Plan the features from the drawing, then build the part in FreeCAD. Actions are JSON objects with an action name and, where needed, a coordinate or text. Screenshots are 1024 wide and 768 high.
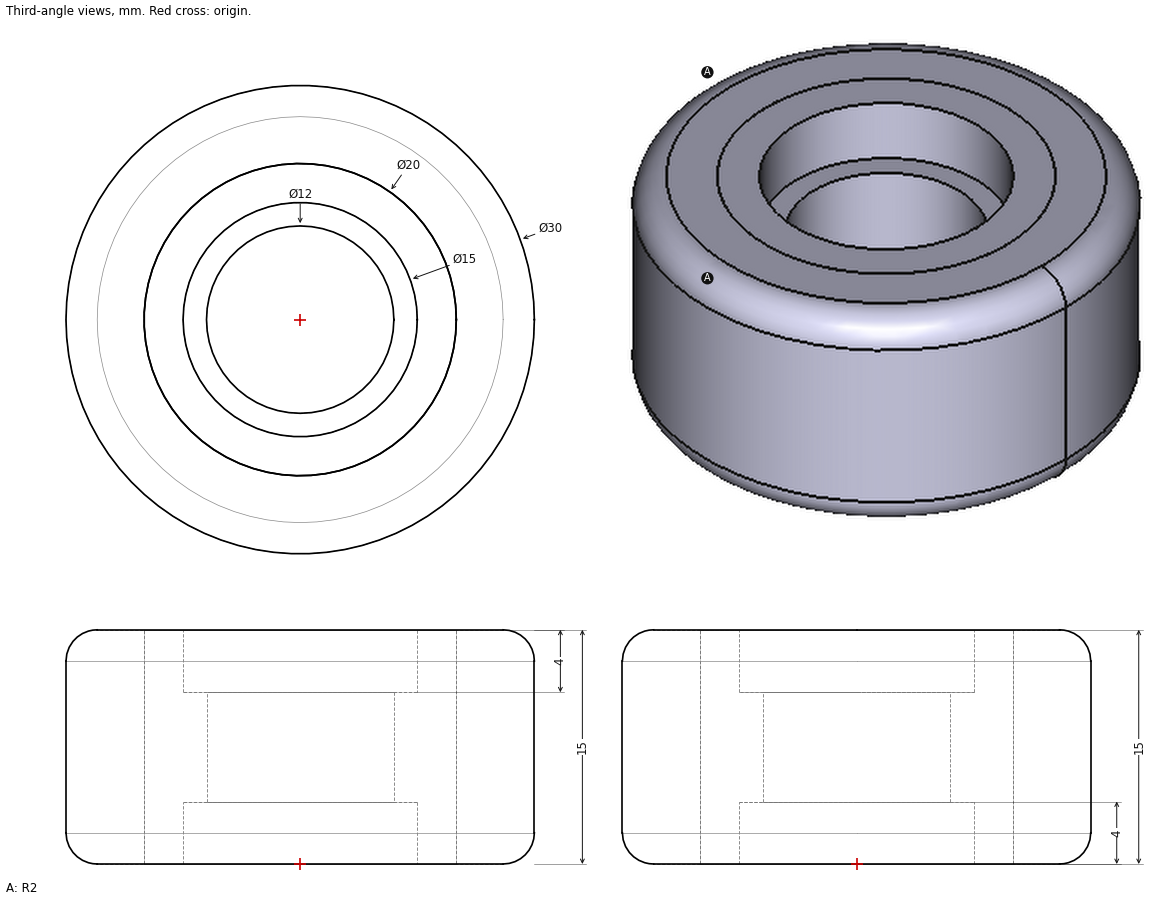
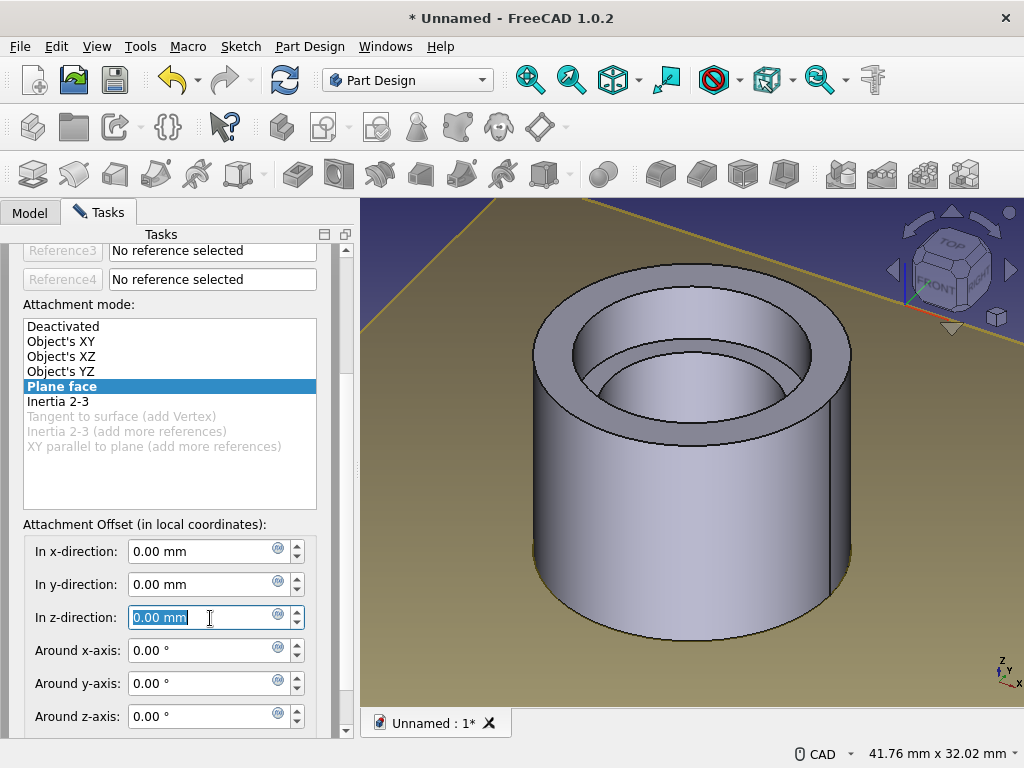
{"action": "type", "text": "15"}
{"action": "key", "text": "Tab"}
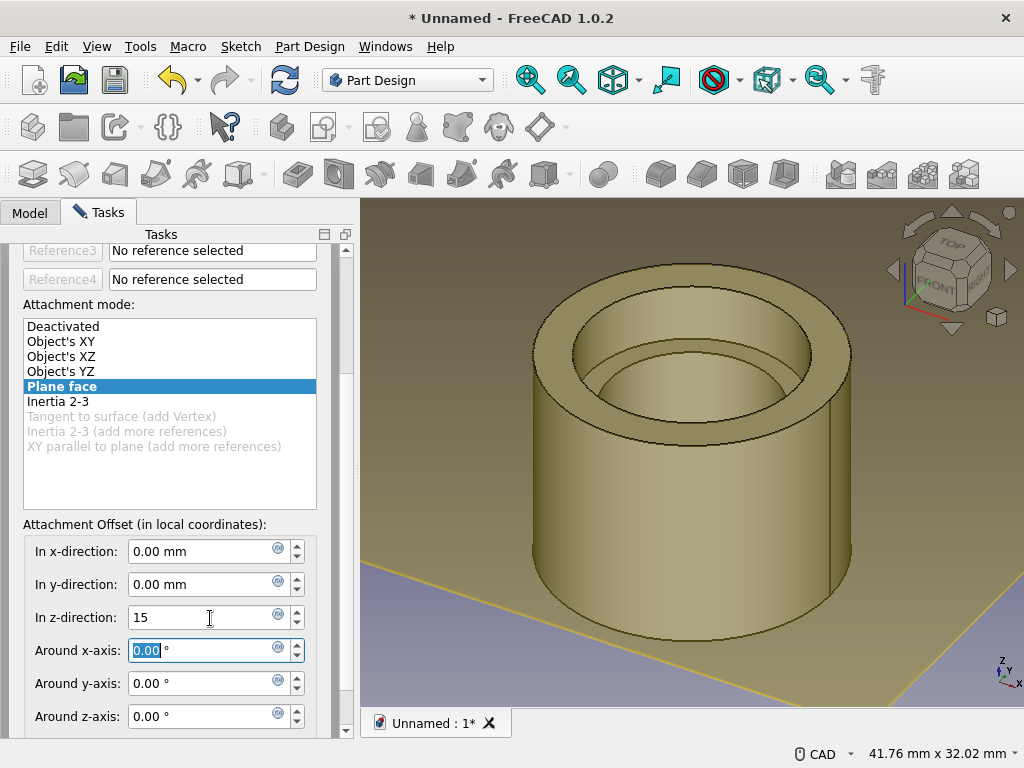
{"action": "scroll", "coordinate": [346, 491], "scroll_direction": "up", "scroll_amount": 4}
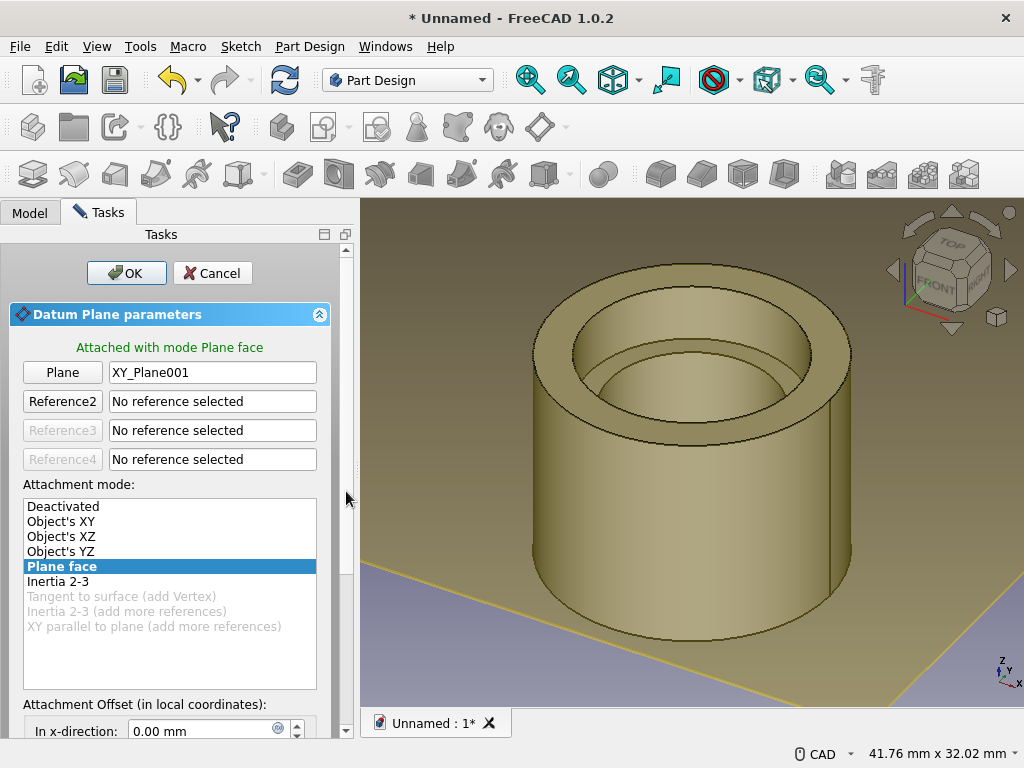
{"action": "left_click", "coordinate": [127, 273]}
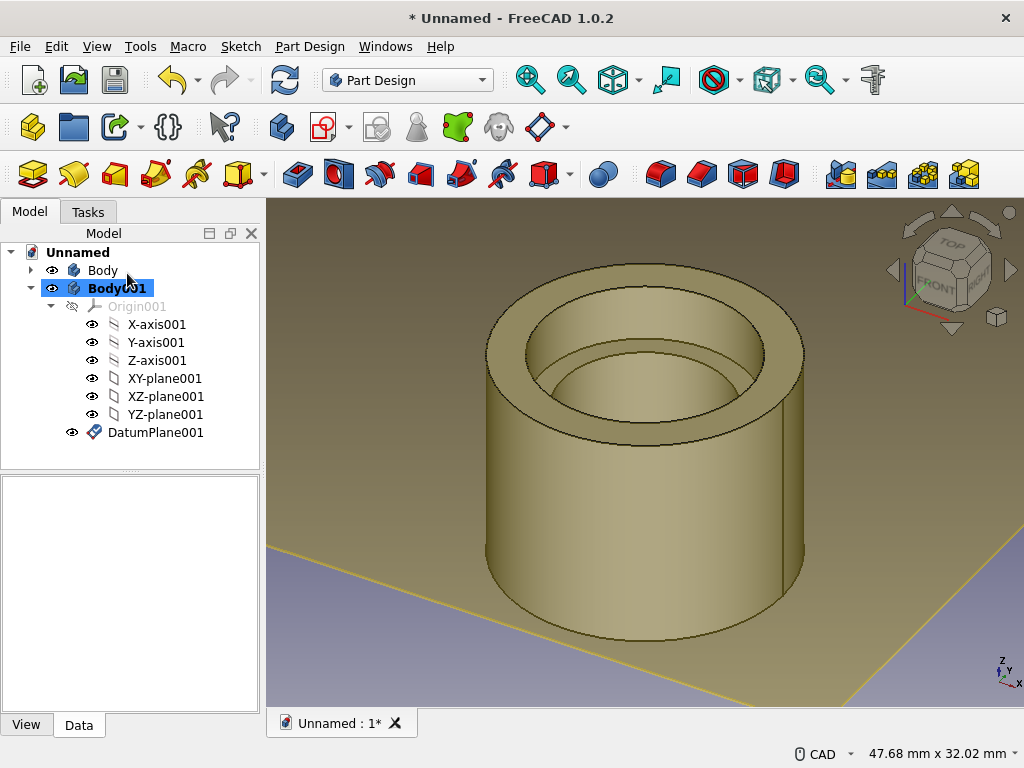
{"action": "left_click", "coordinate": [117, 432]}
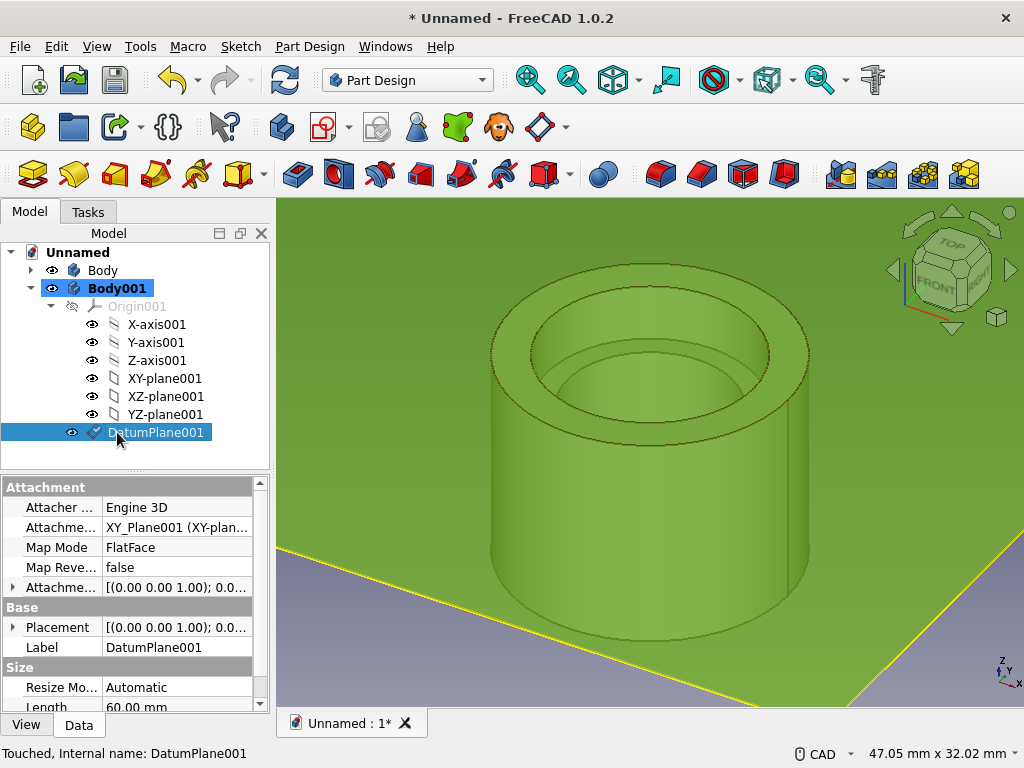
{"action": "left_click", "coordinate": [322, 128]}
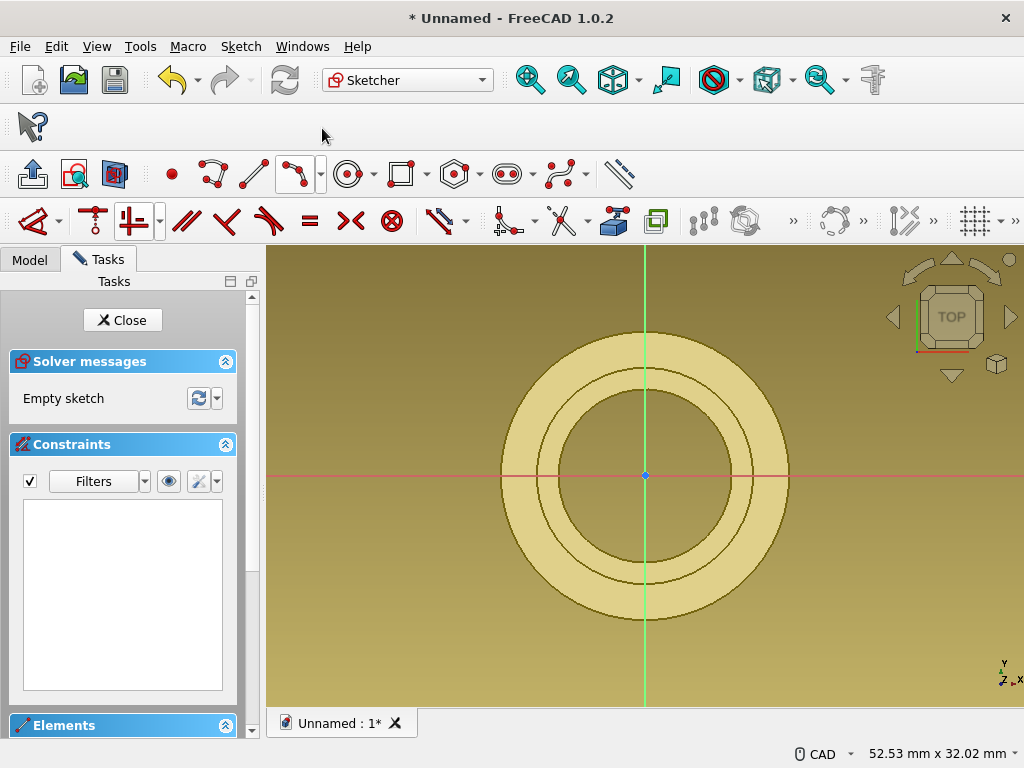
{"action": "scroll", "coordinate": [437, 476], "scroll_direction": "down", "scroll_amount": 2}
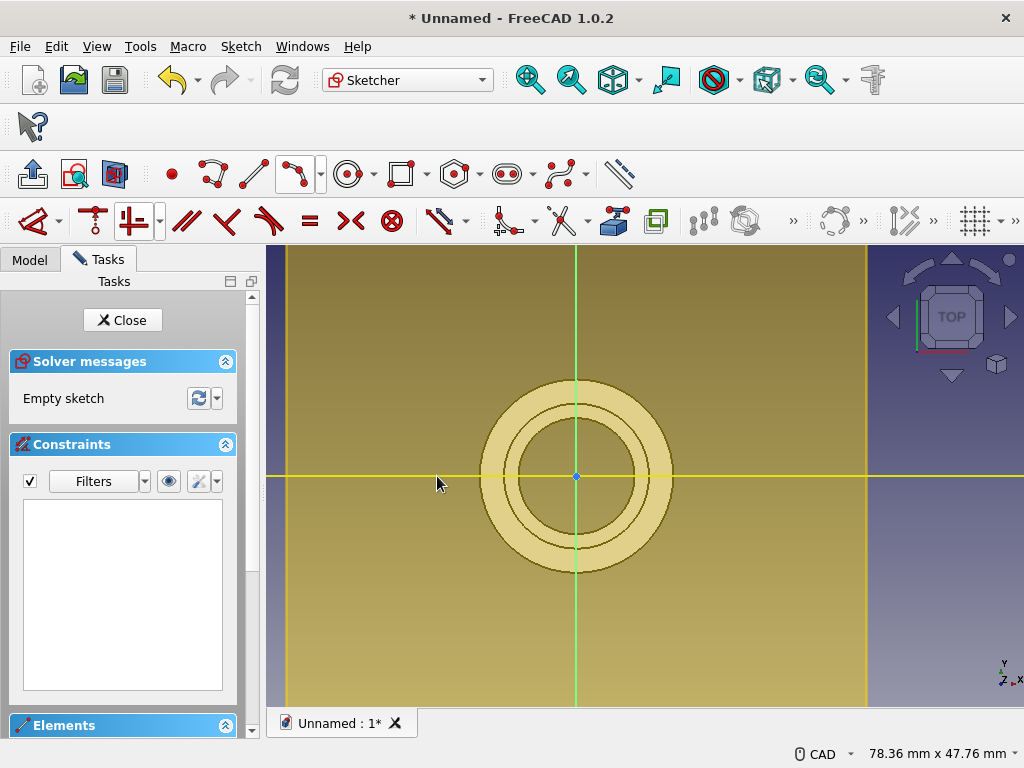
{"action": "left_click", "coordinate": [348, 174]}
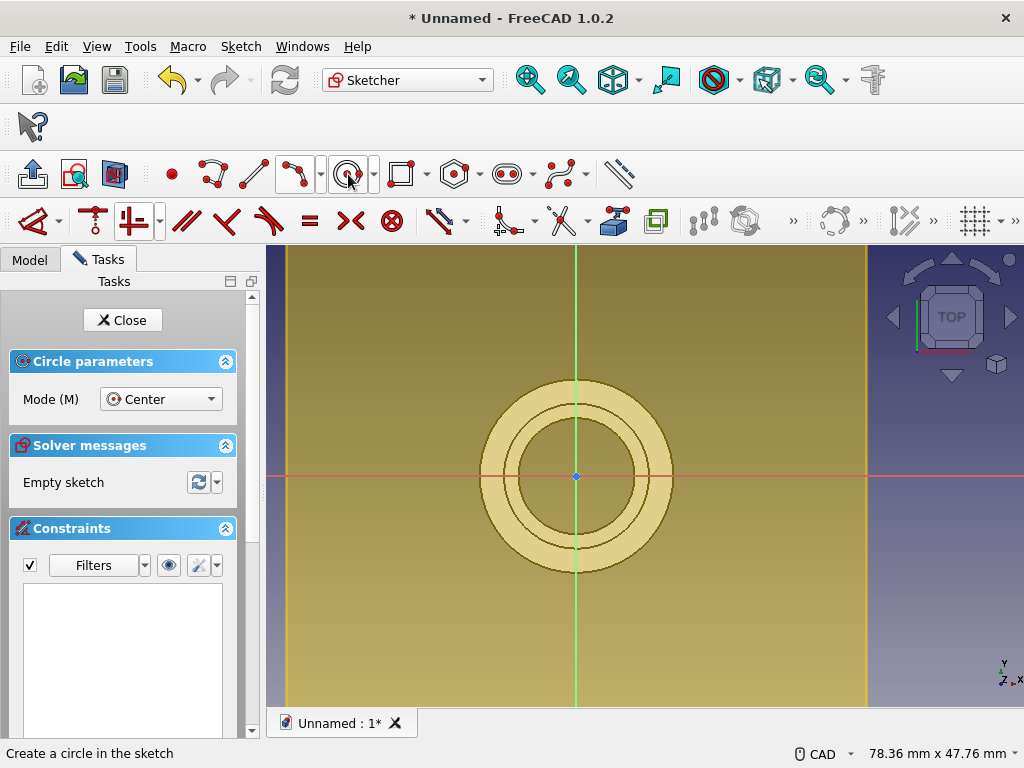
{"action": "left_click", "coordinate": [577, 476]}
{"action": "mouse_move", "coordinate": [679, 374]}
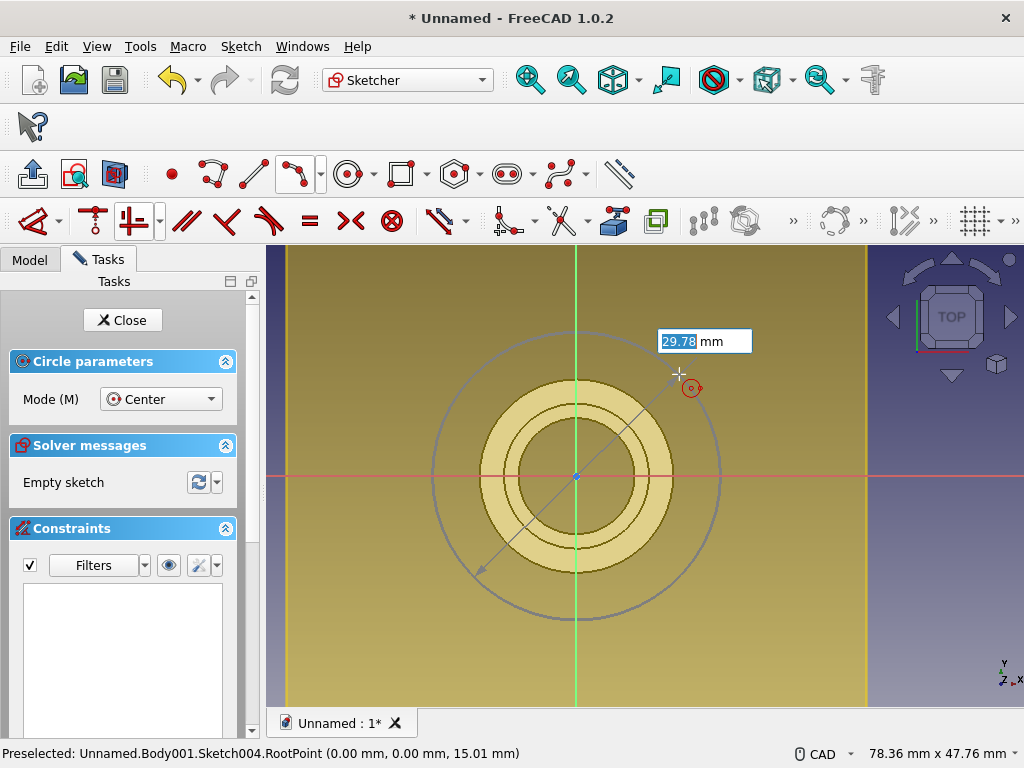
{"action": "type", "text": "30"}
{"action": "key", "text": "Return"}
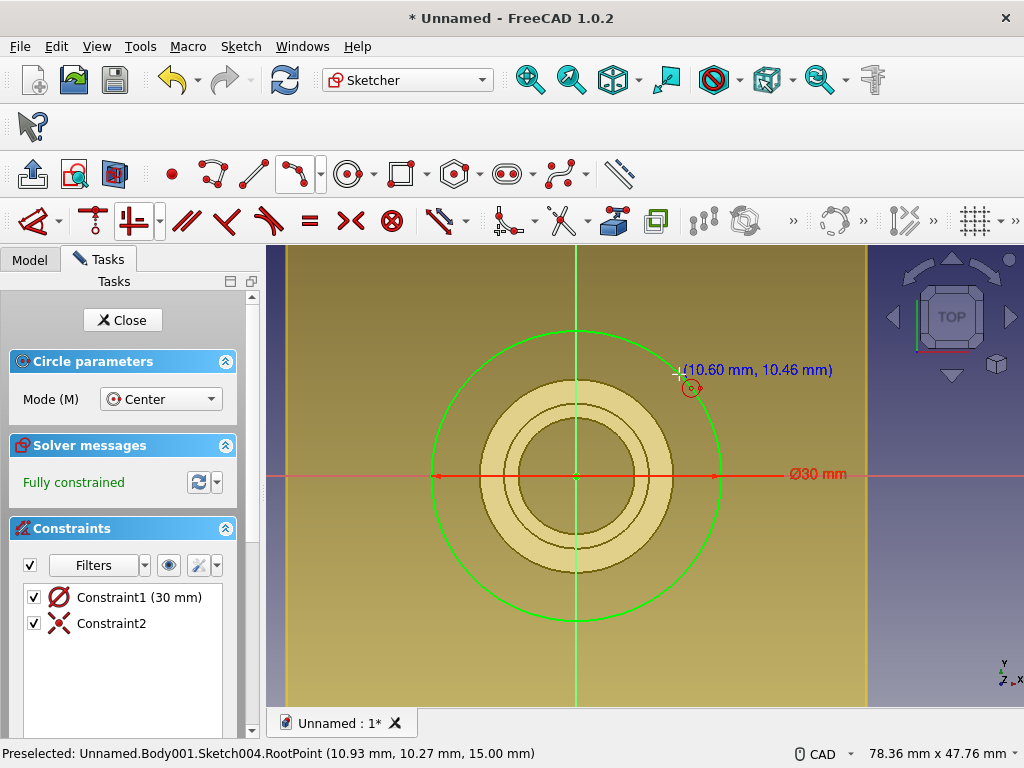
{"action": "left_click", "coordinate": [577, 476]}
{"action": "mouse_move", "coordinate": [645, 408]}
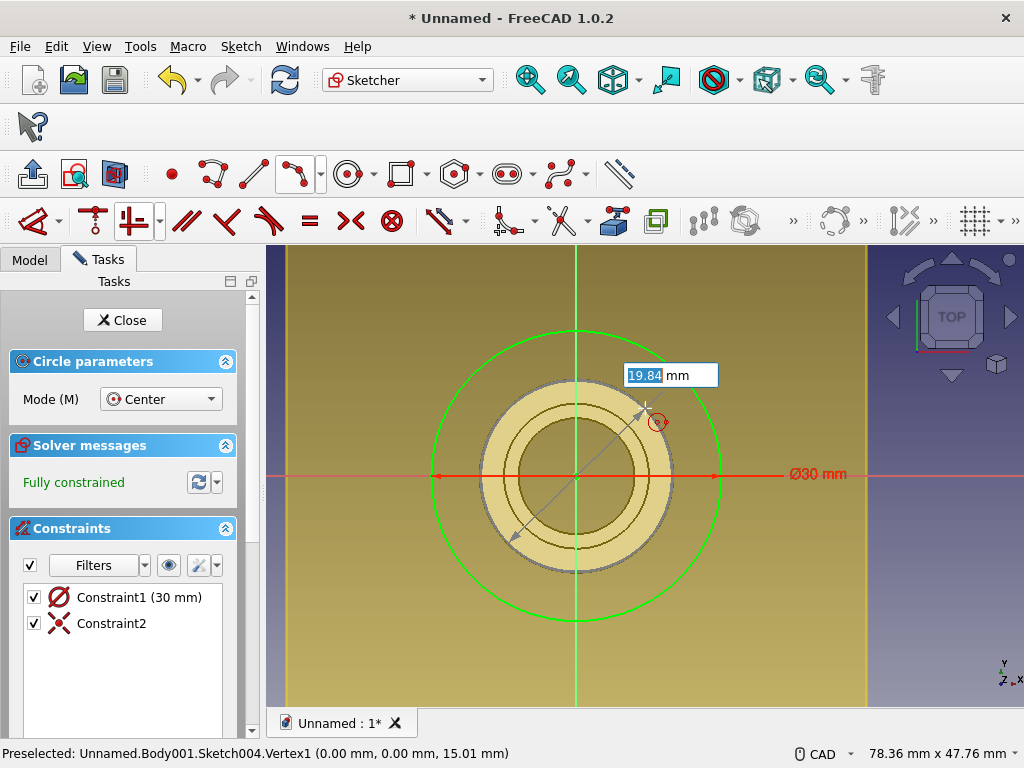
{"action": "type", "text": "20"}
{"action": "key", "text": "Return"}
{"action": "key", "text": "Escape"}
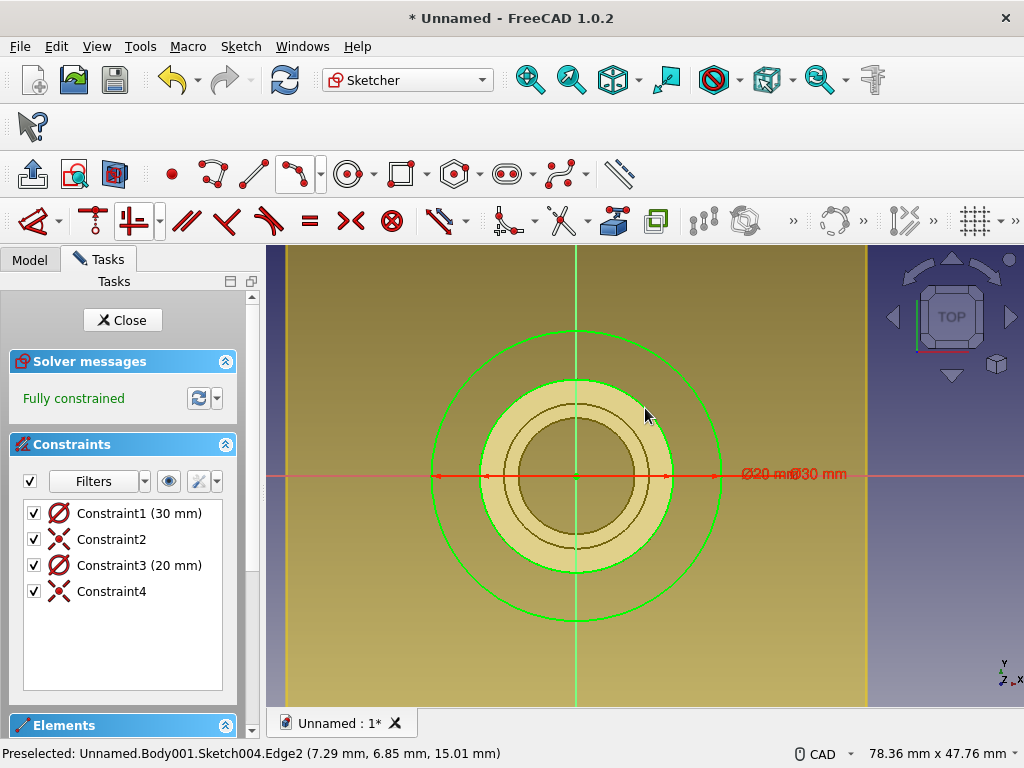
{"action": "left_click", "coordinate": [123, 320]}